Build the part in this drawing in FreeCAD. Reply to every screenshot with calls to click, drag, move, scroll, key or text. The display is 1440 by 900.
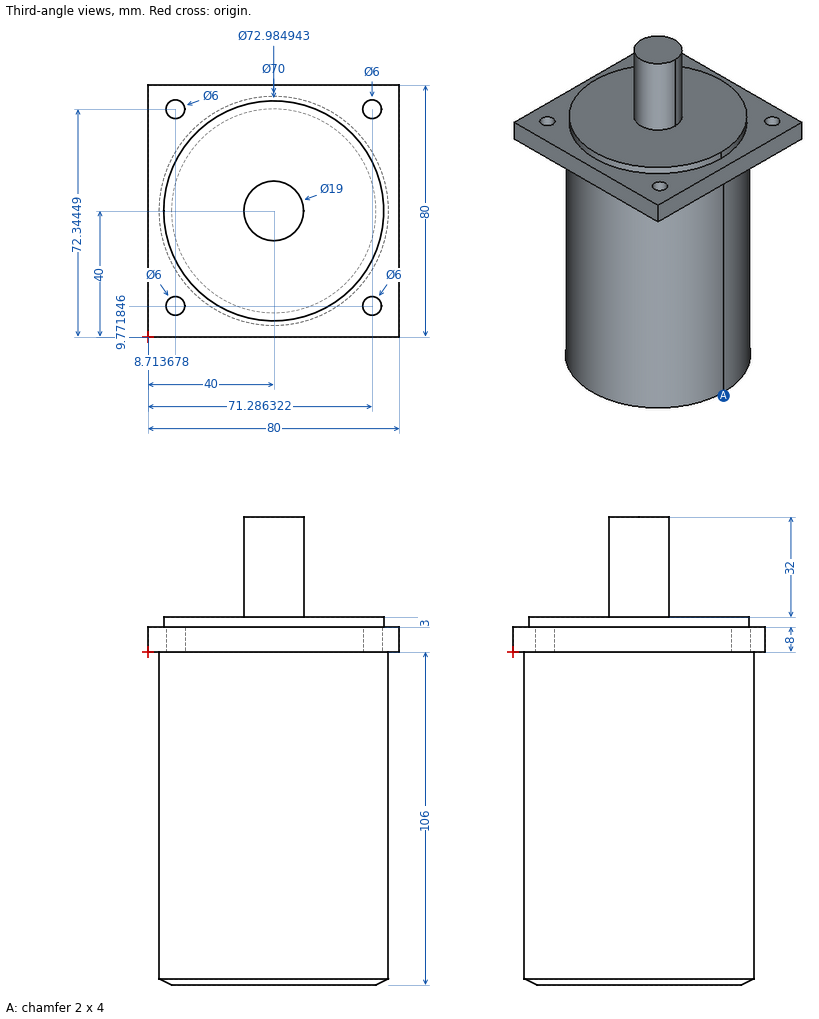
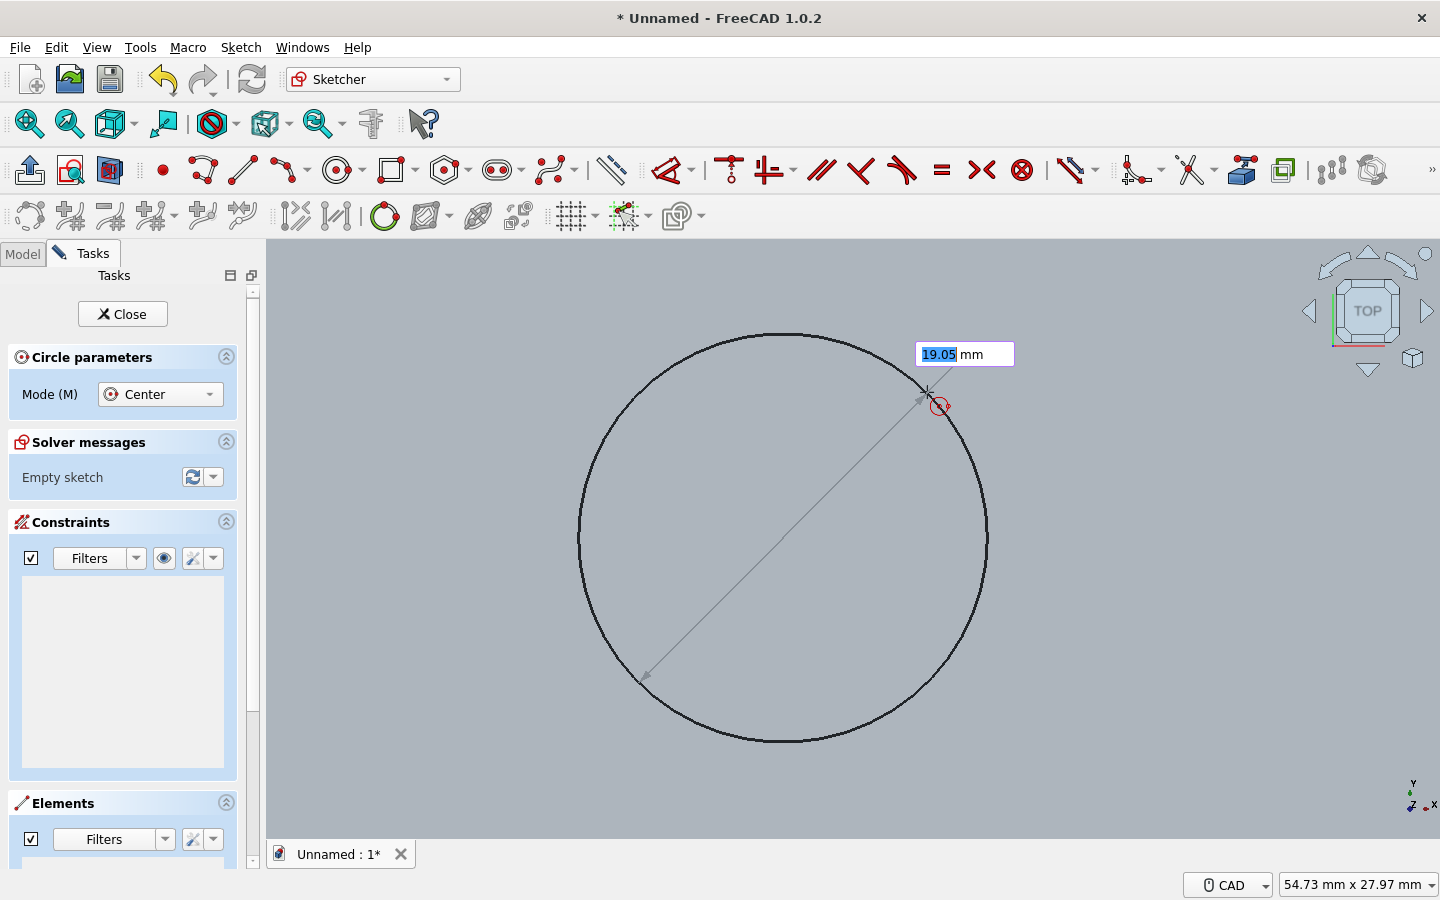
text(19)
key(Return)
key(Escape)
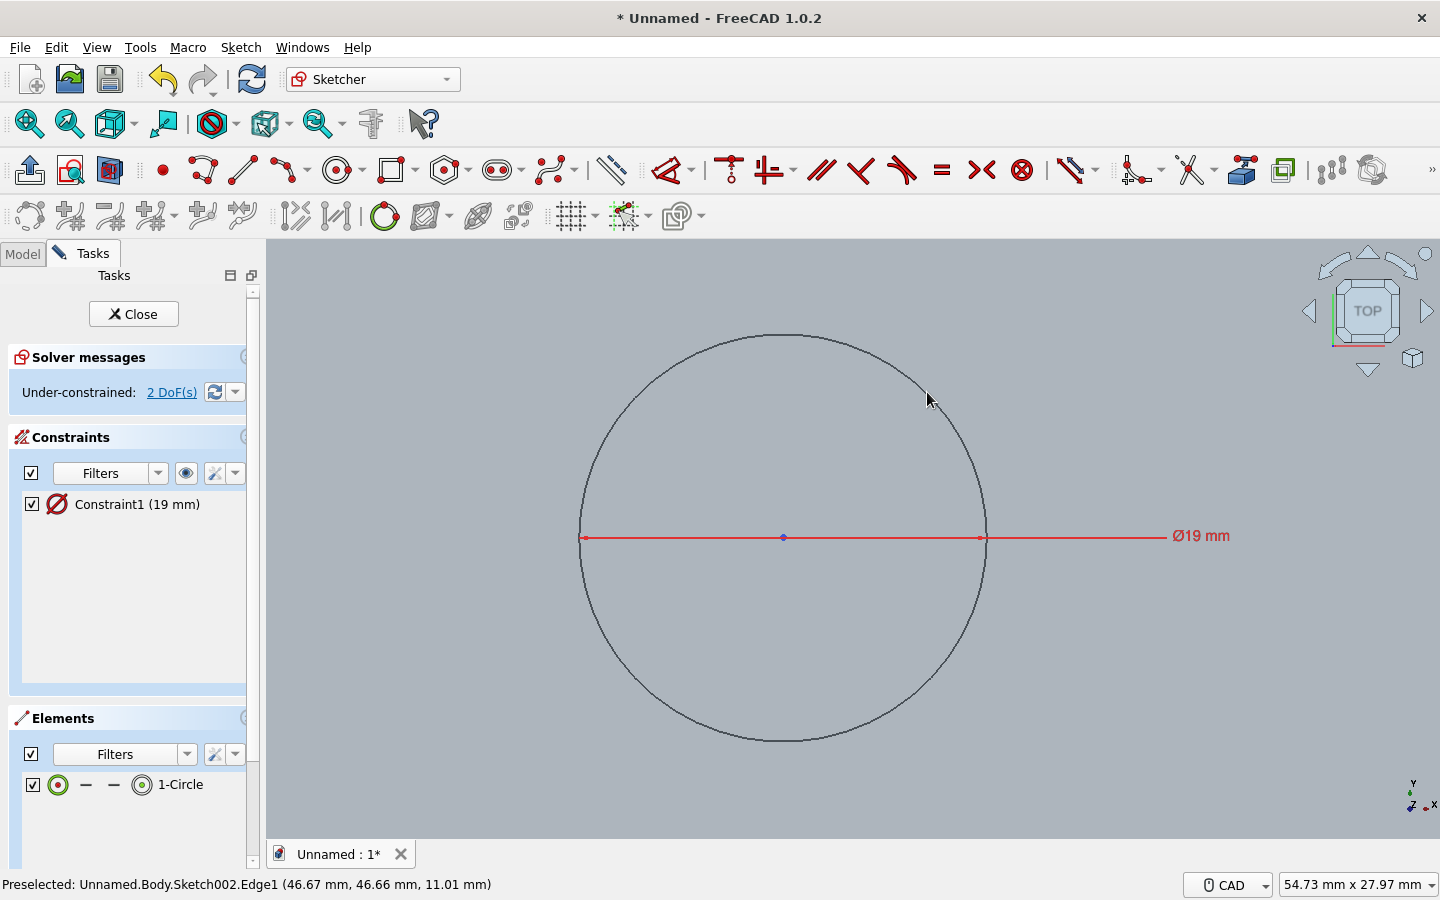
click(666, 170)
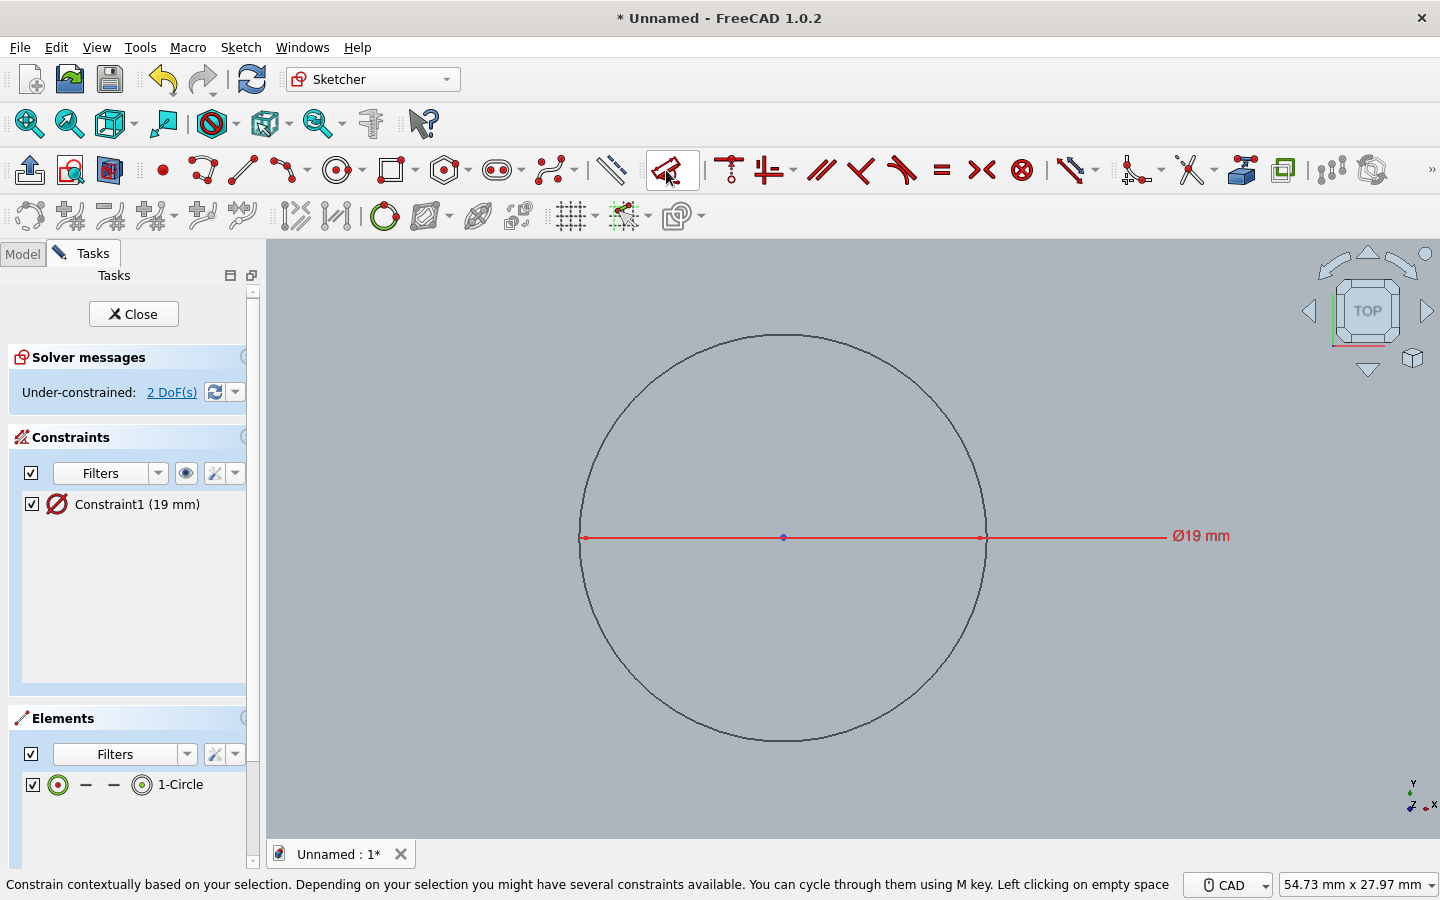
click(783, 538)
click(538, 504)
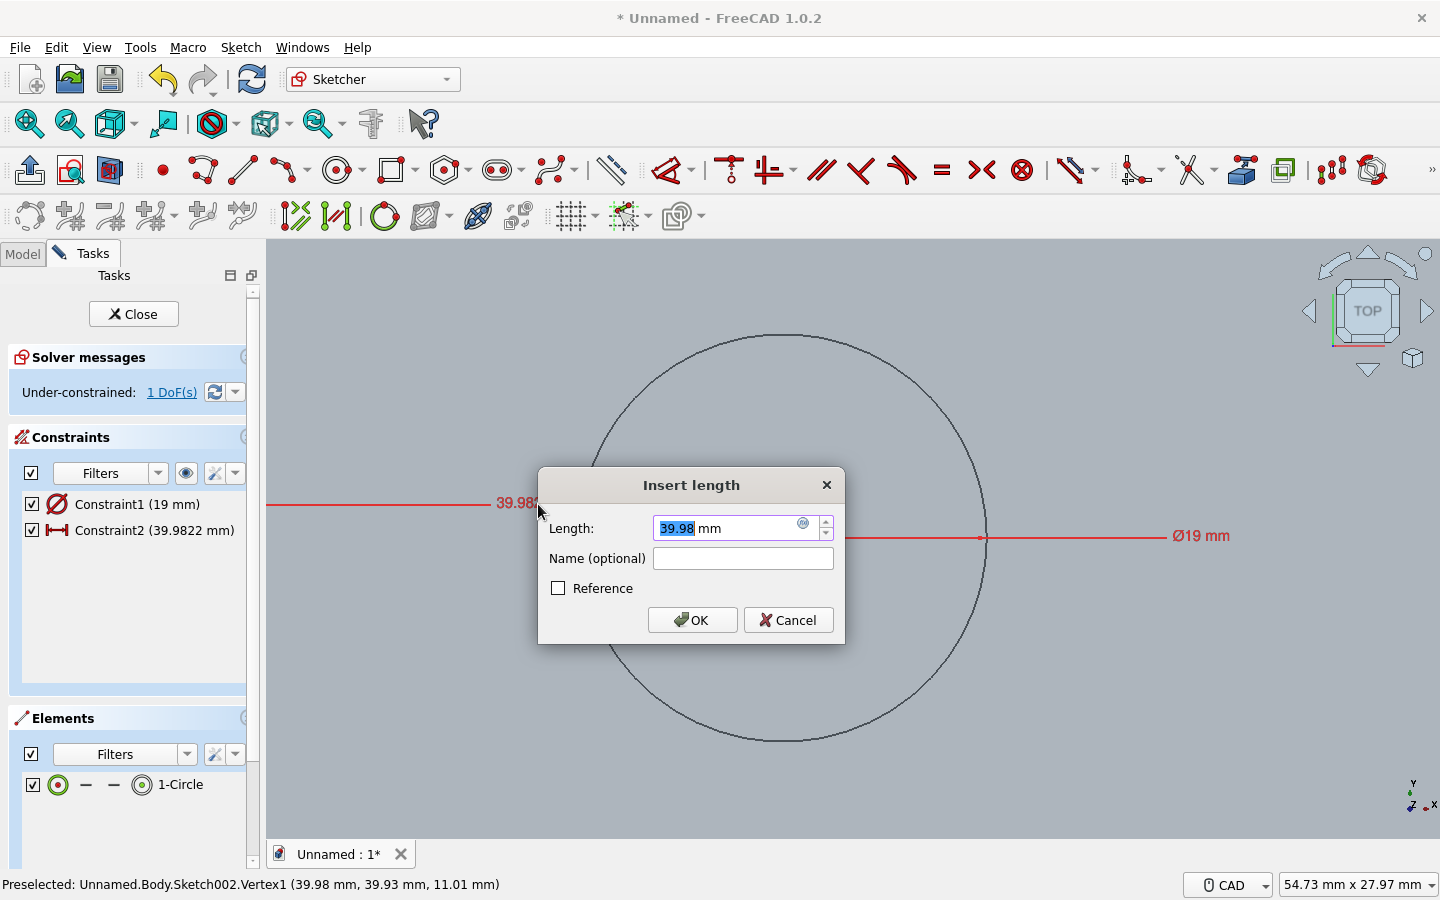
text(40)
key(Return)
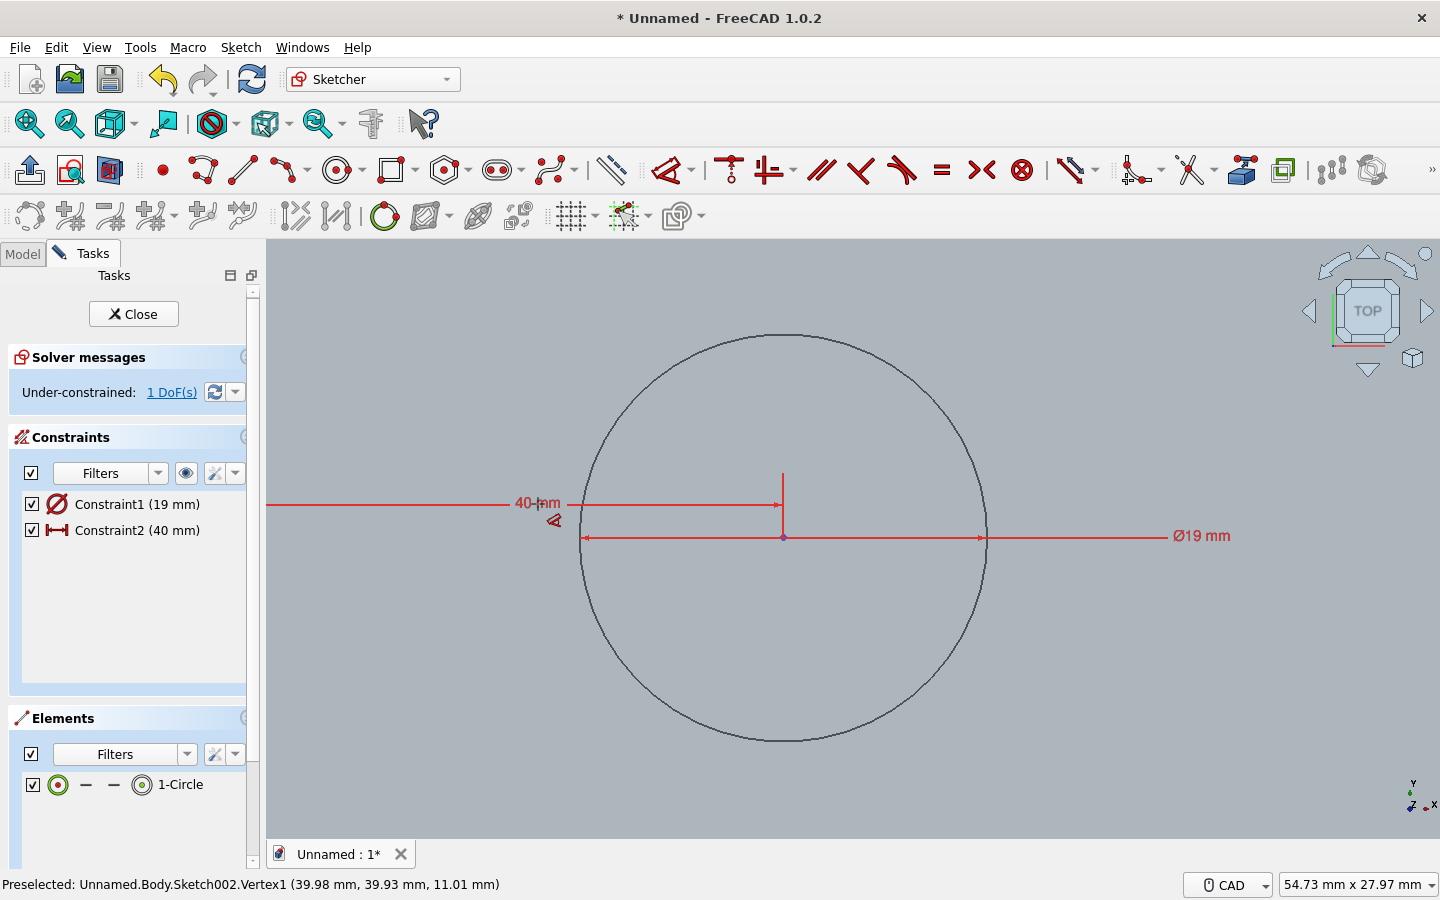
click(783, 538)
click(817, 674)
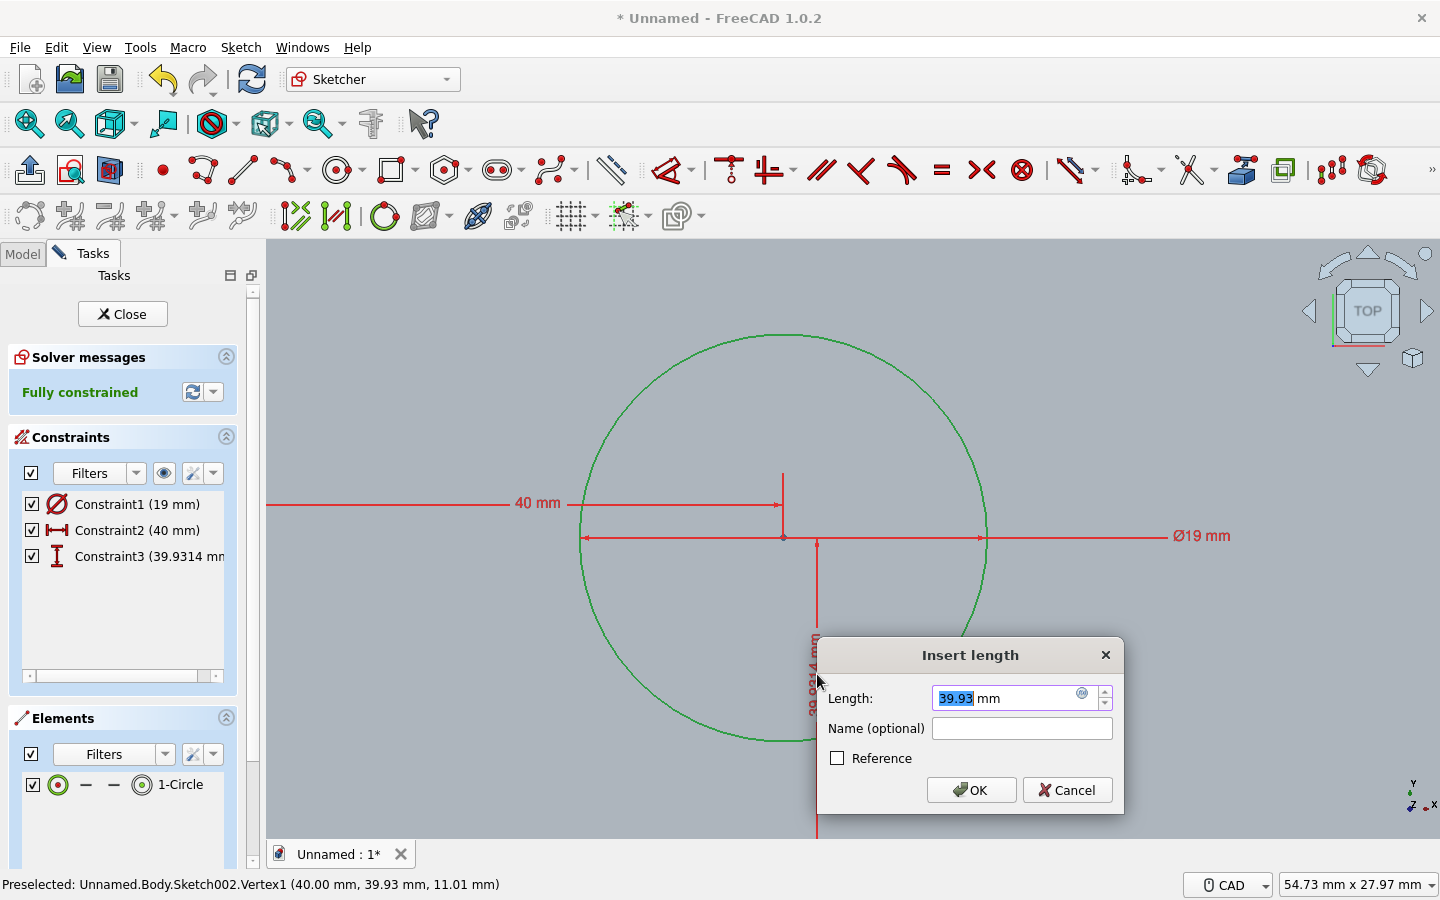
text(40)
key(Return)
key(Escape)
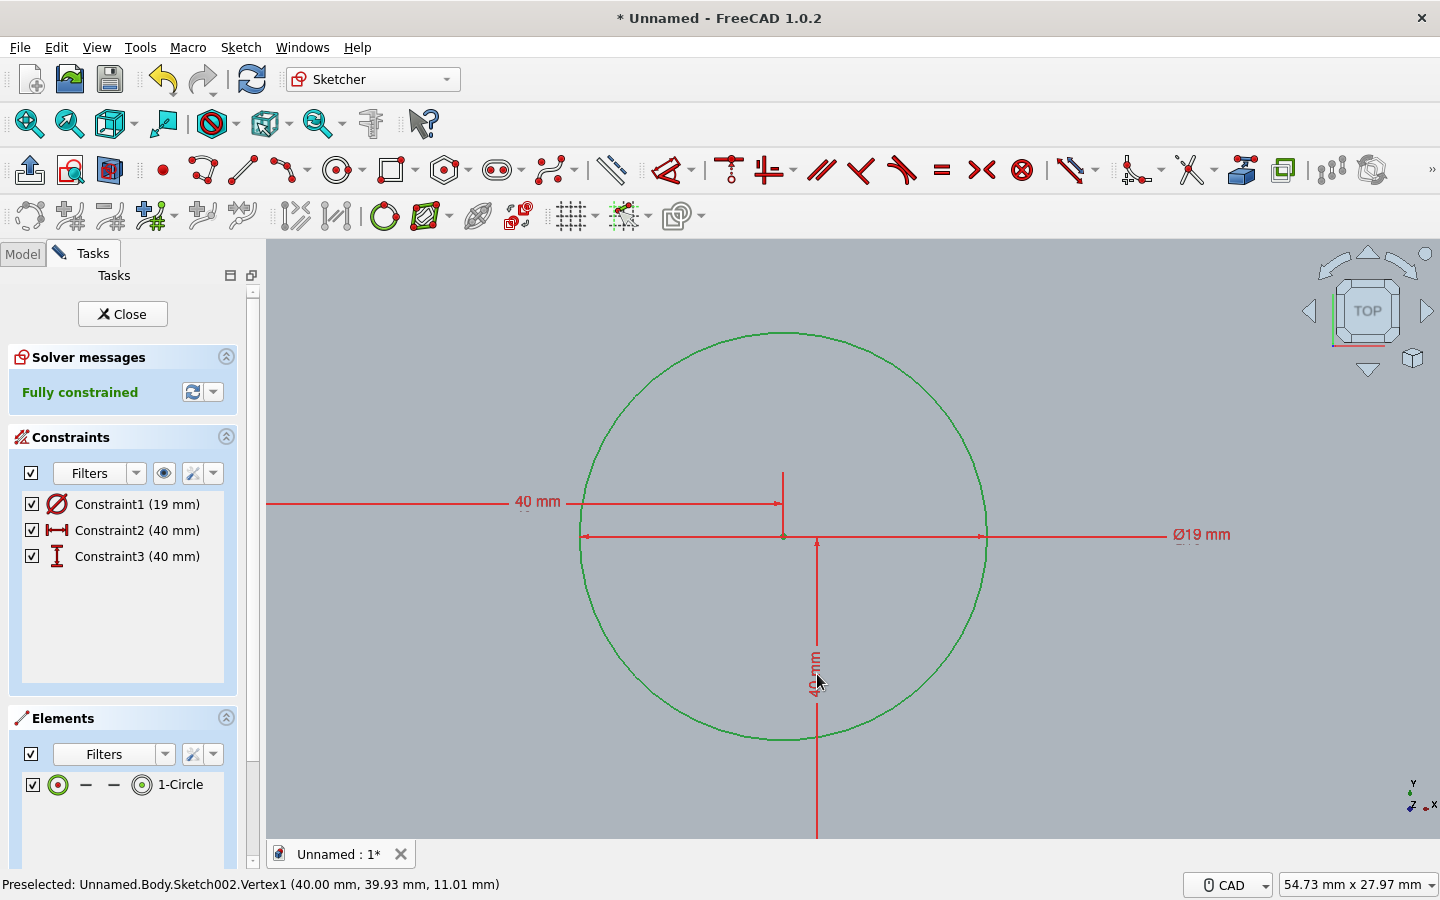
click(123, 314)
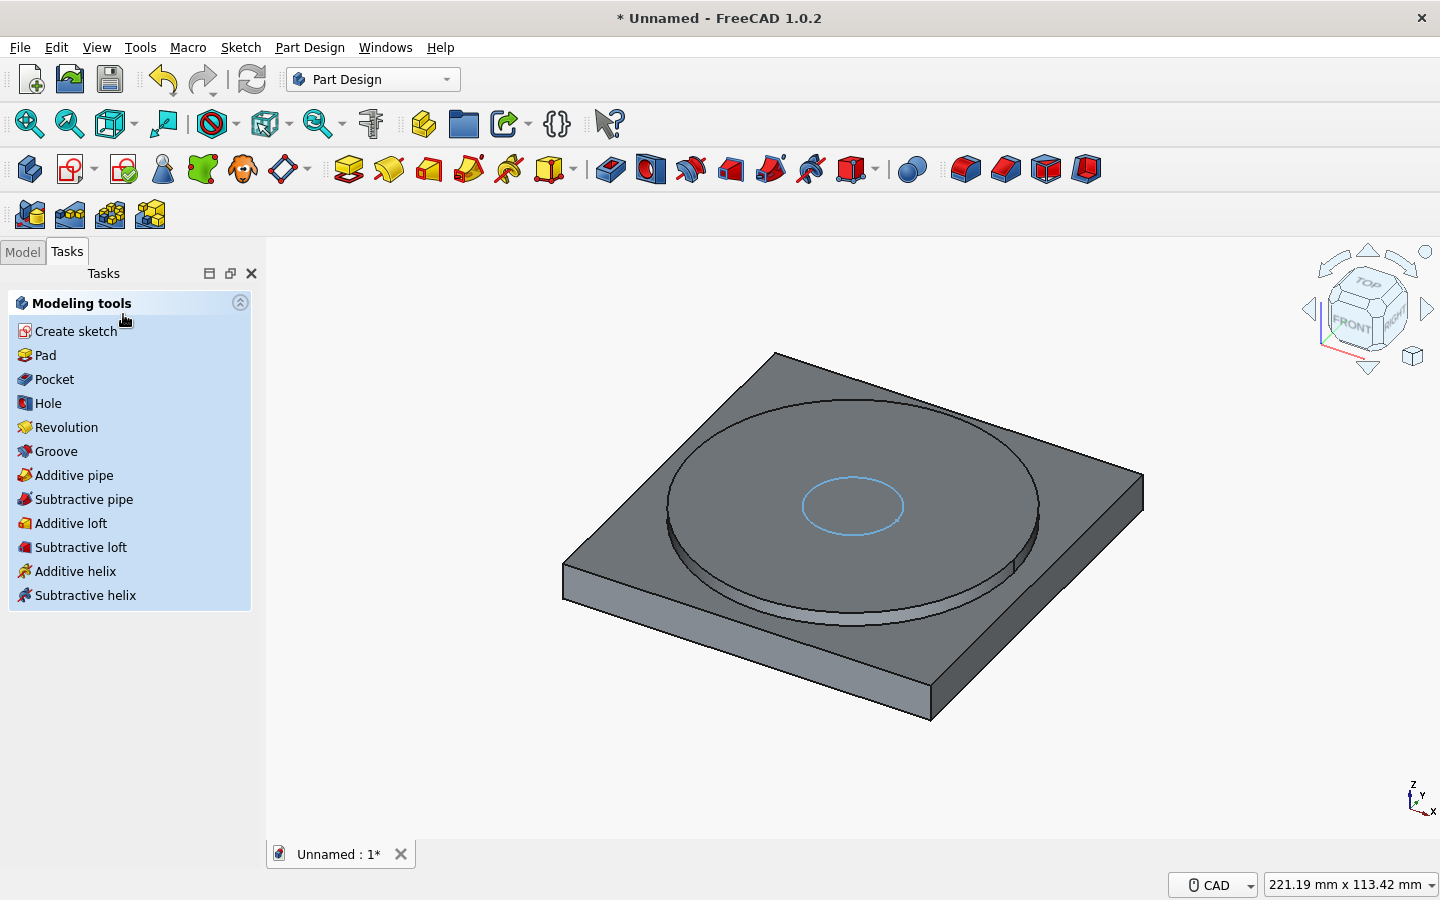
click(350, 170)